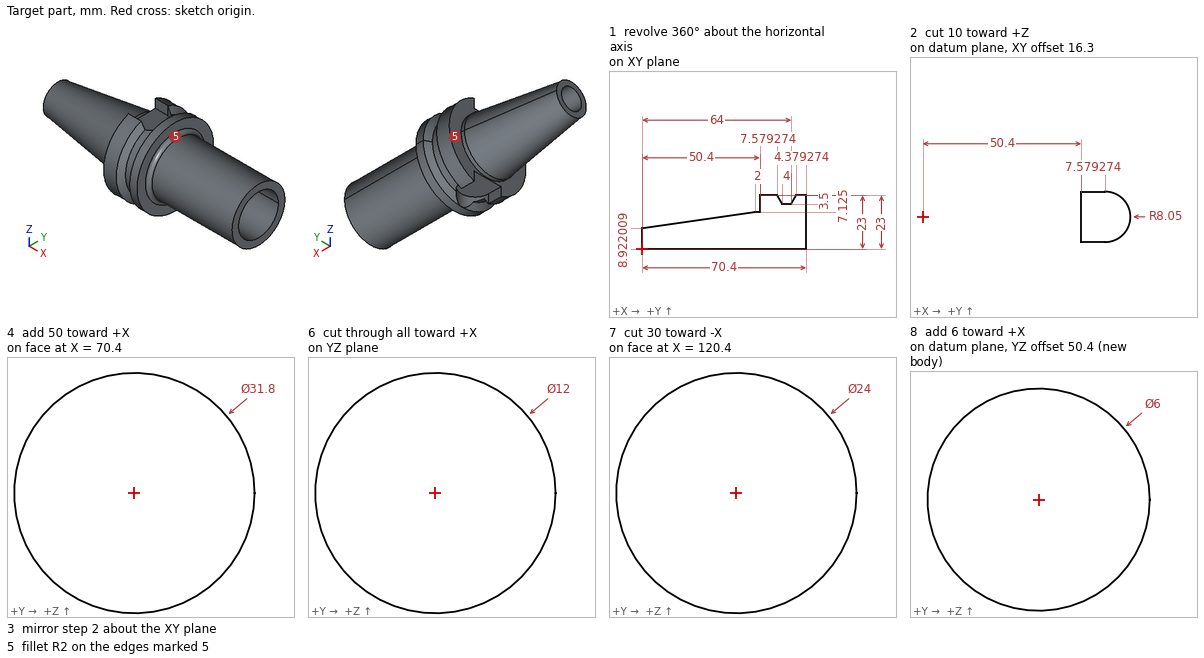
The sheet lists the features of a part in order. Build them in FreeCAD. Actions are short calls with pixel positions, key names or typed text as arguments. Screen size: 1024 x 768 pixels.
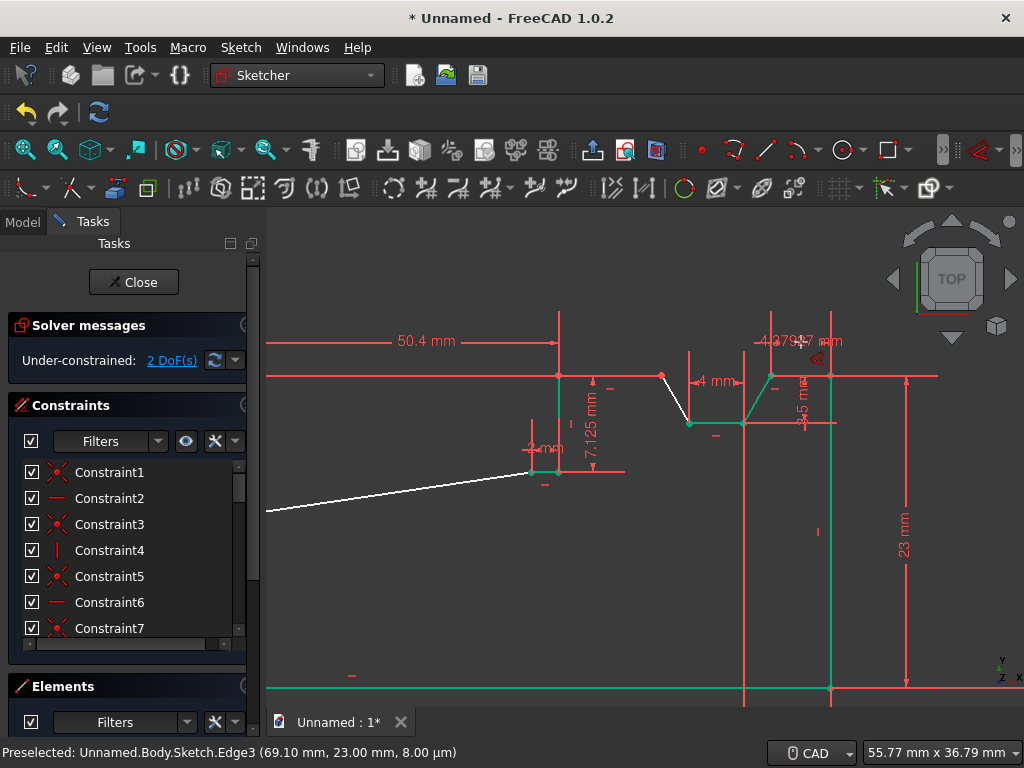
click(631, 376)
click(610, 342)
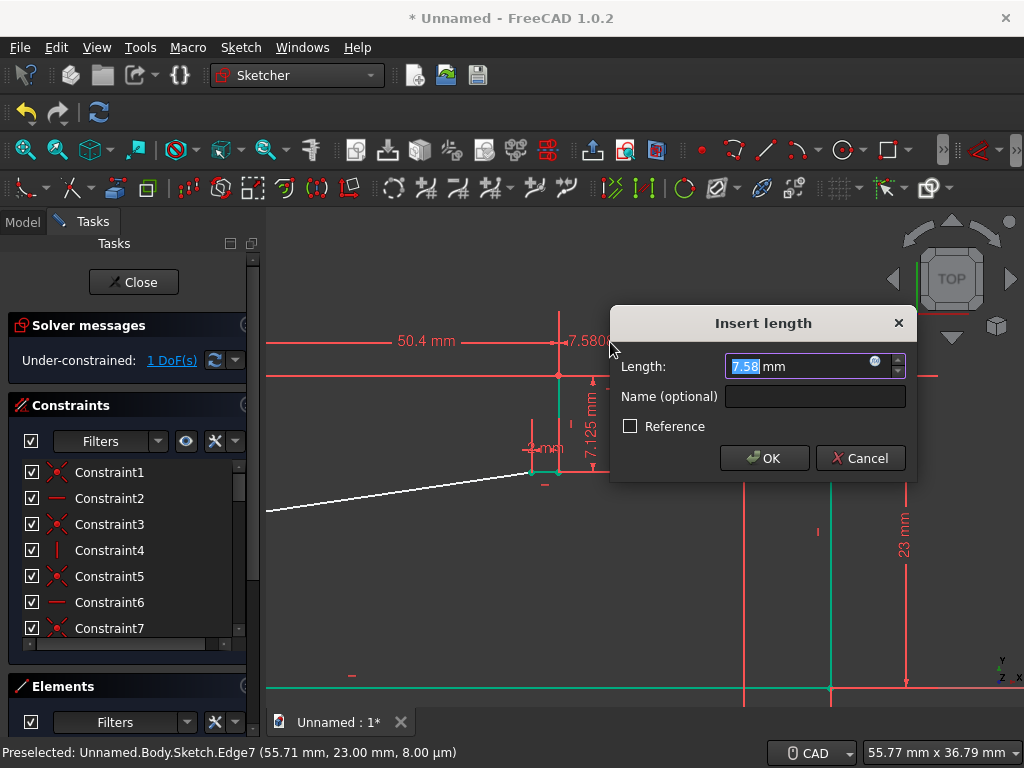
text(7.579274)
key(Return)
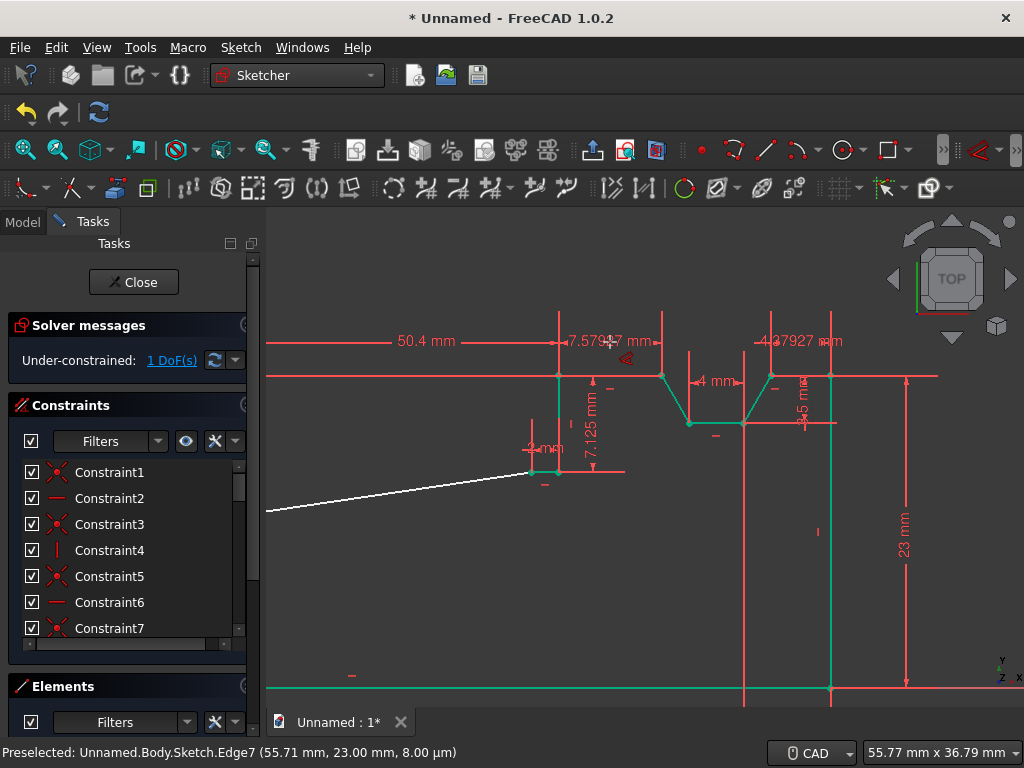
scroll(759, 396, down, 4)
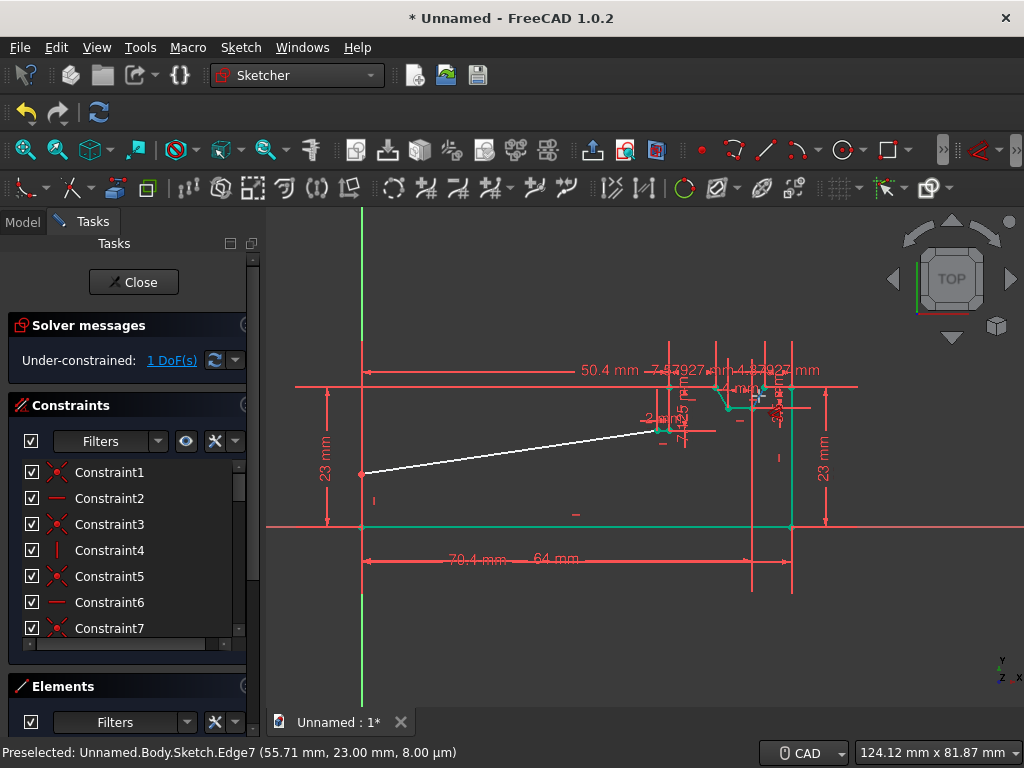
click(362, 490)
click(328, 501)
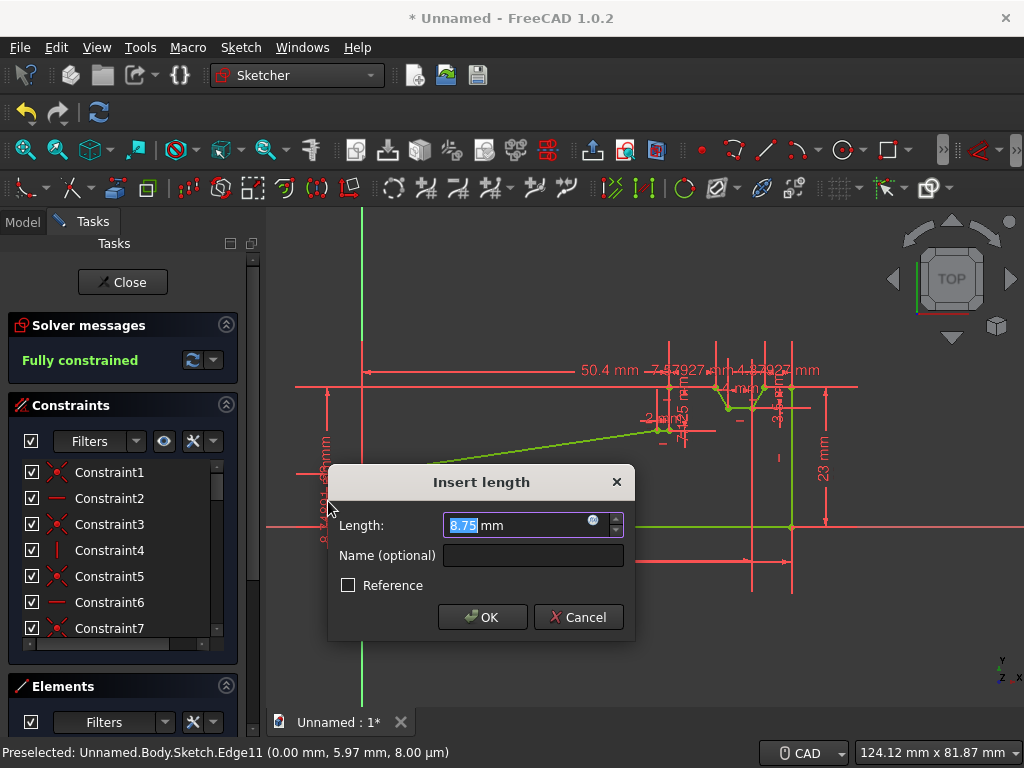
text(8.922009)
key(Return)
key(Escape)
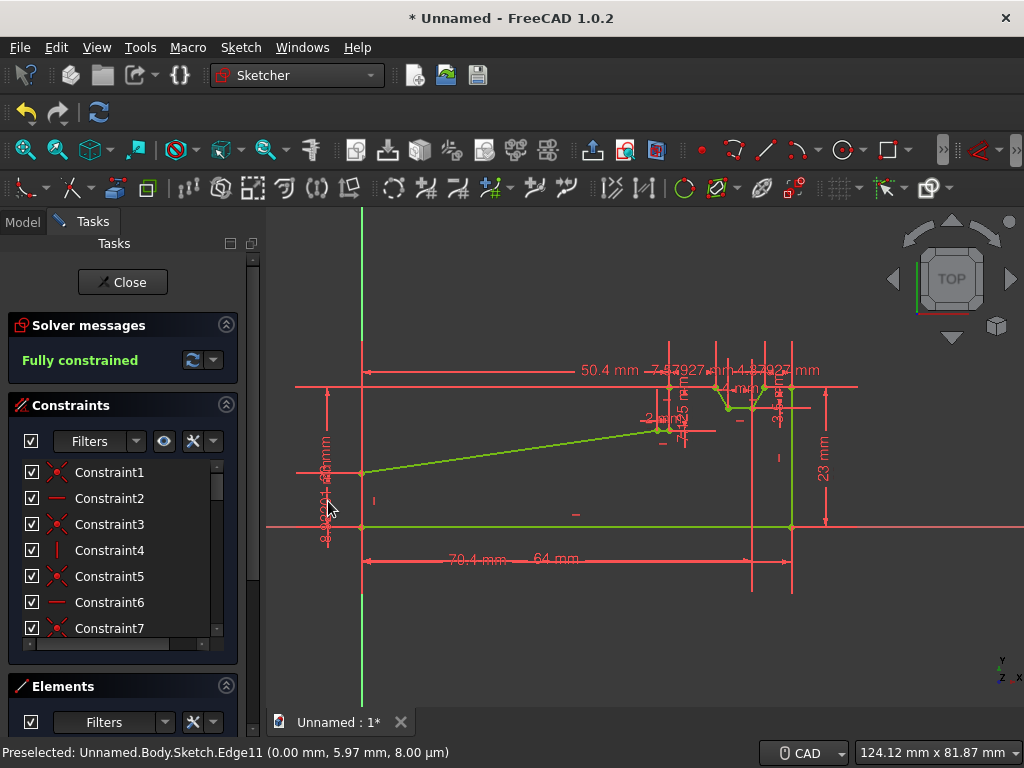
click(123, 282)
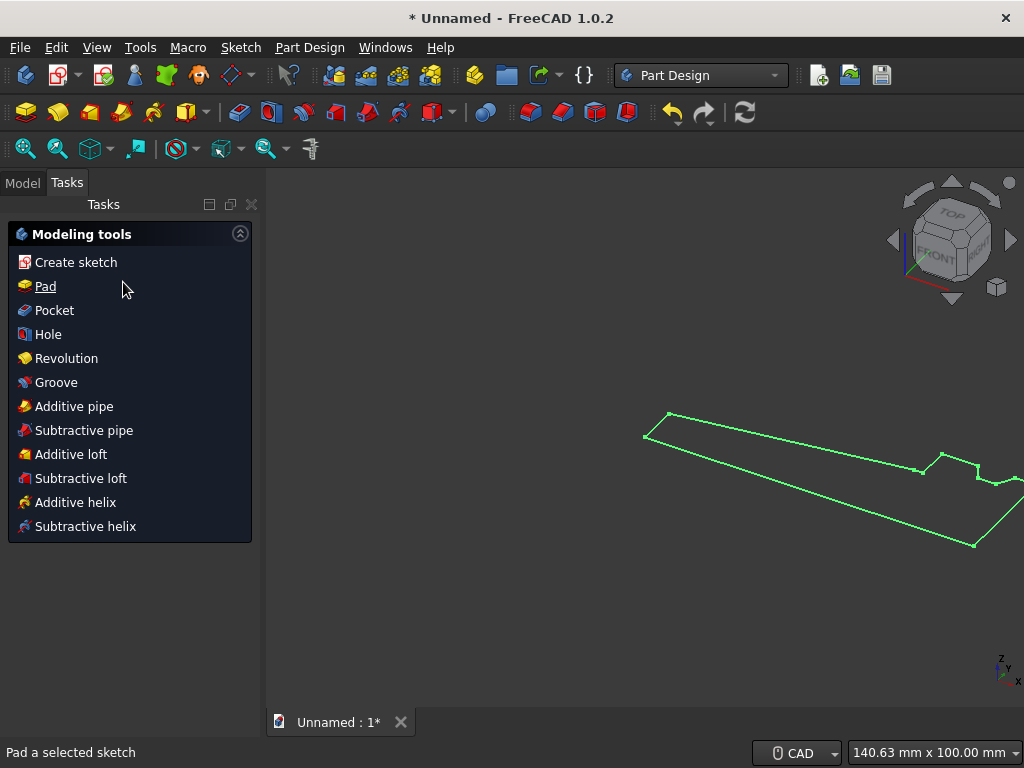
click(58, 112)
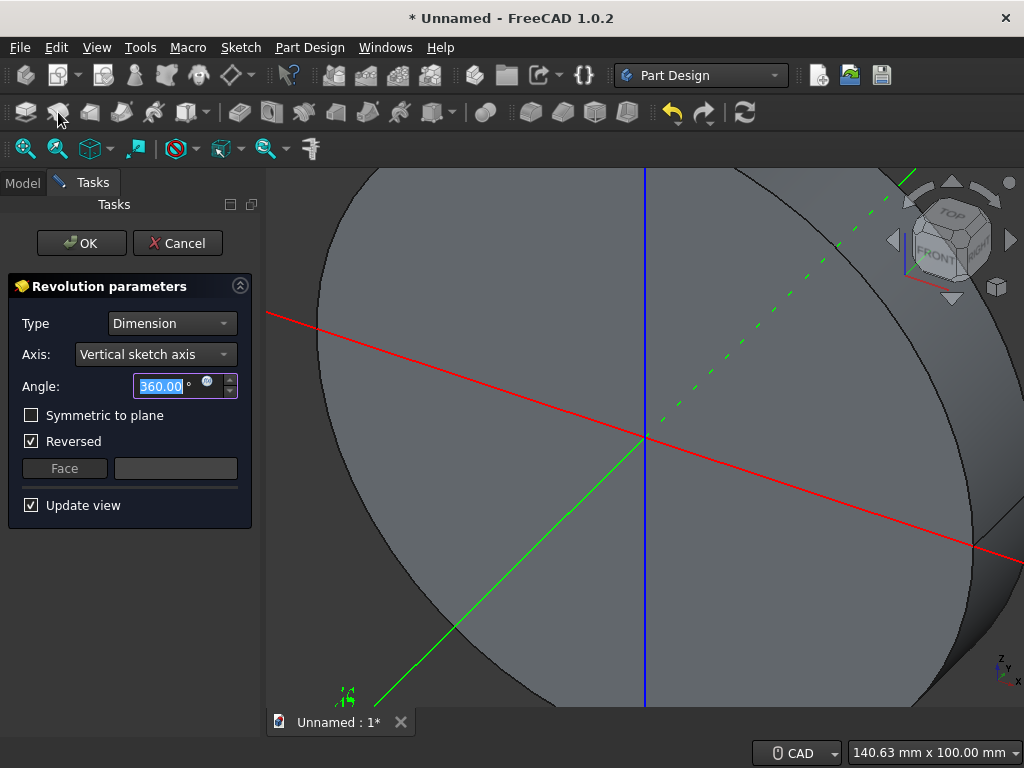
click(156, 354)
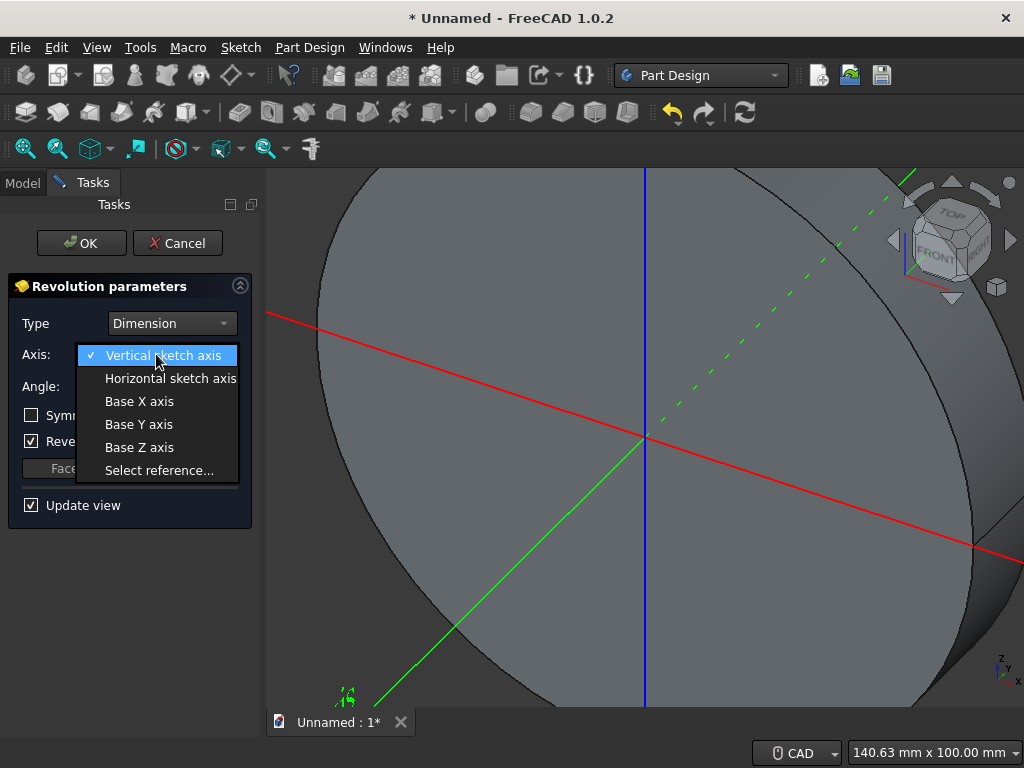
click(156, 378)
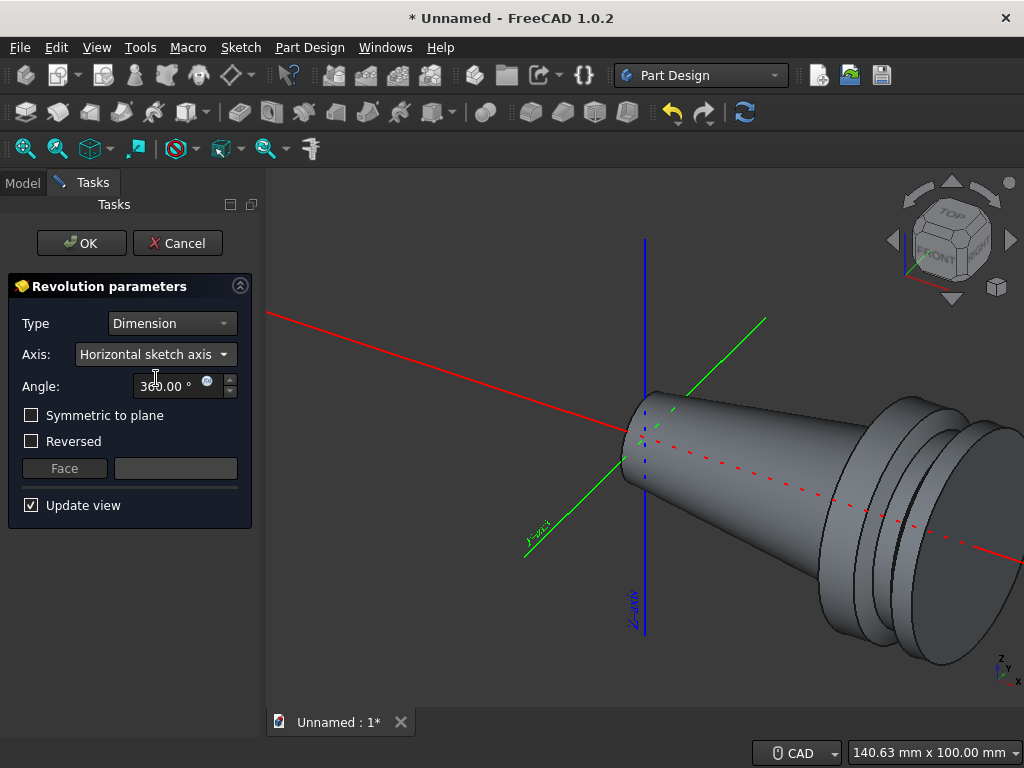
click(82, 243)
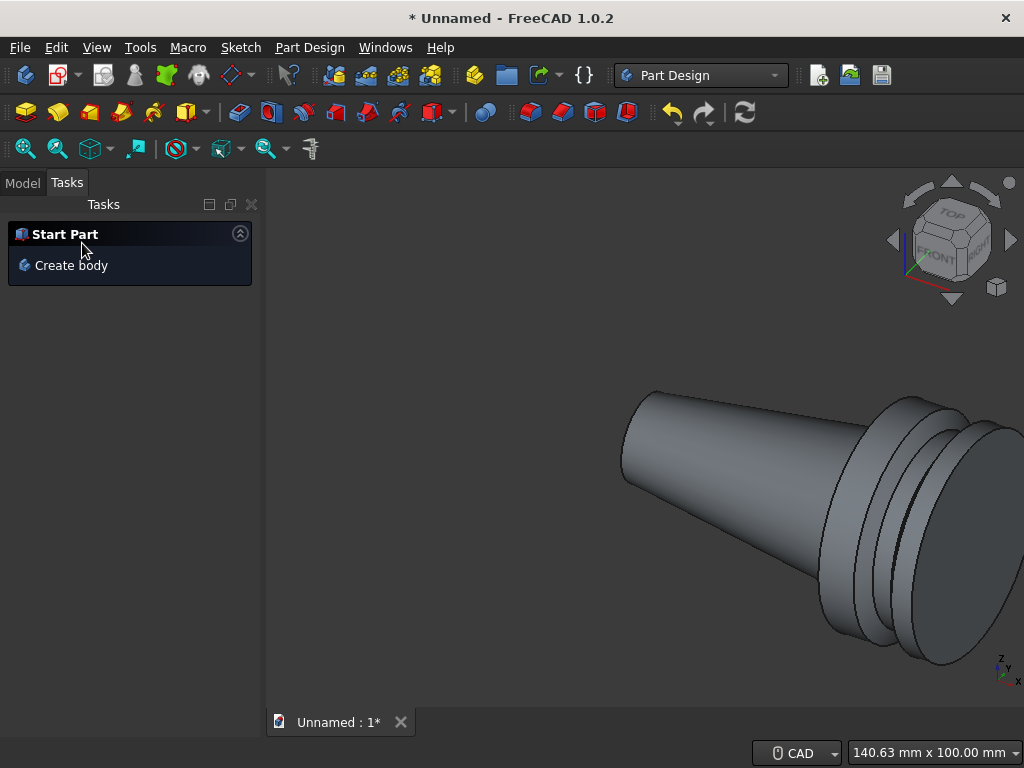
click(26, 150)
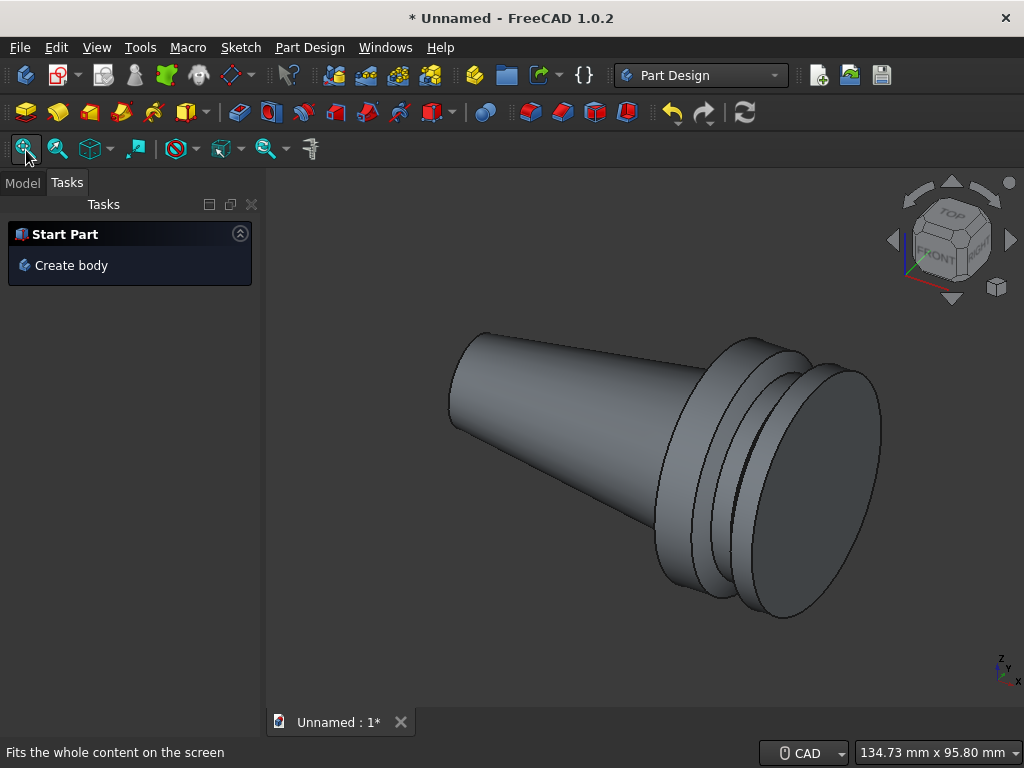
click(23, 182)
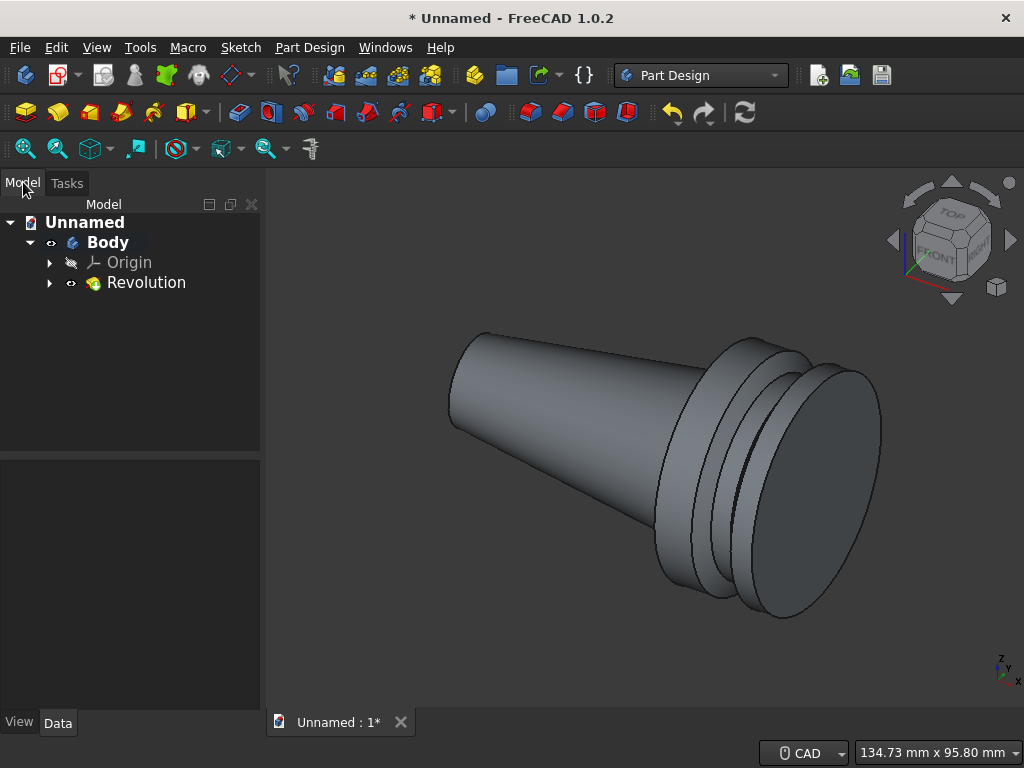
click(50, 263)